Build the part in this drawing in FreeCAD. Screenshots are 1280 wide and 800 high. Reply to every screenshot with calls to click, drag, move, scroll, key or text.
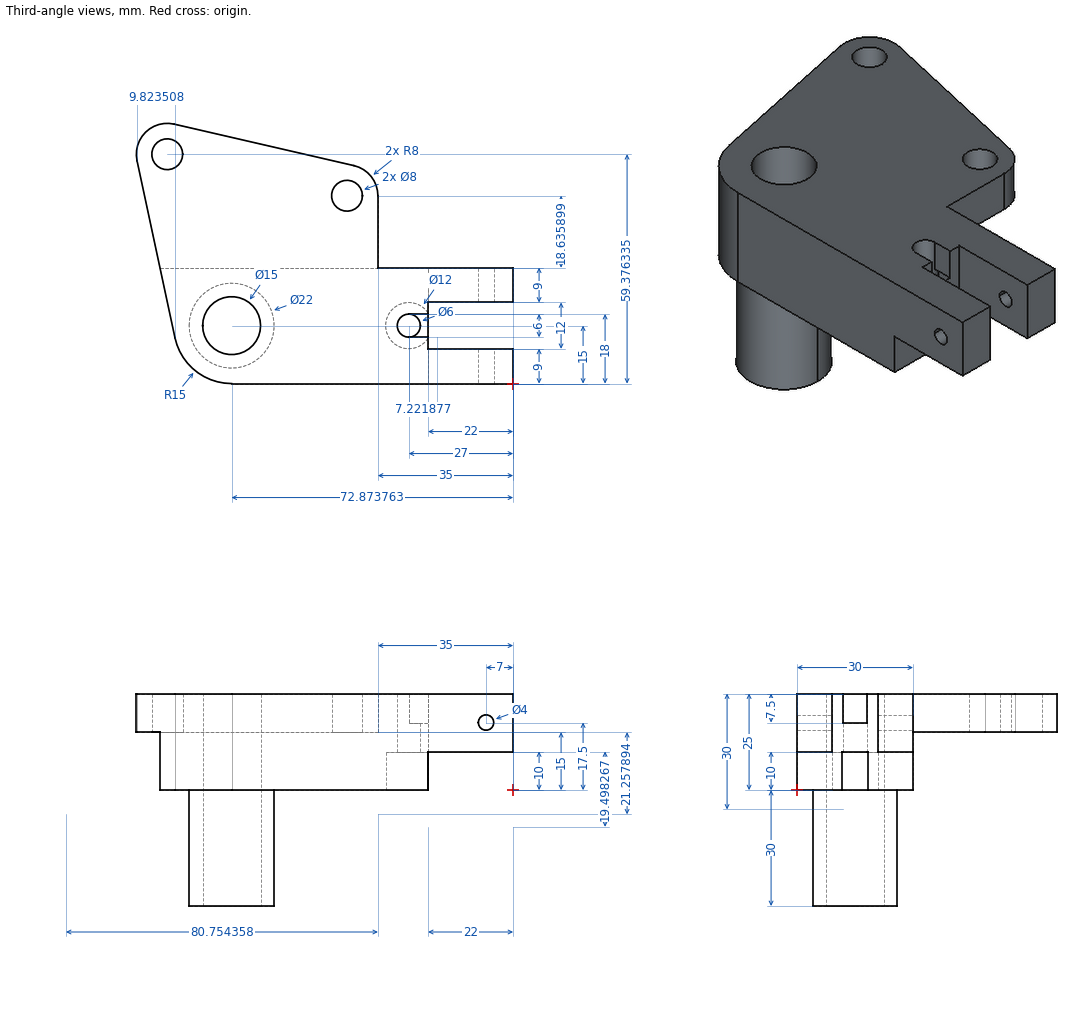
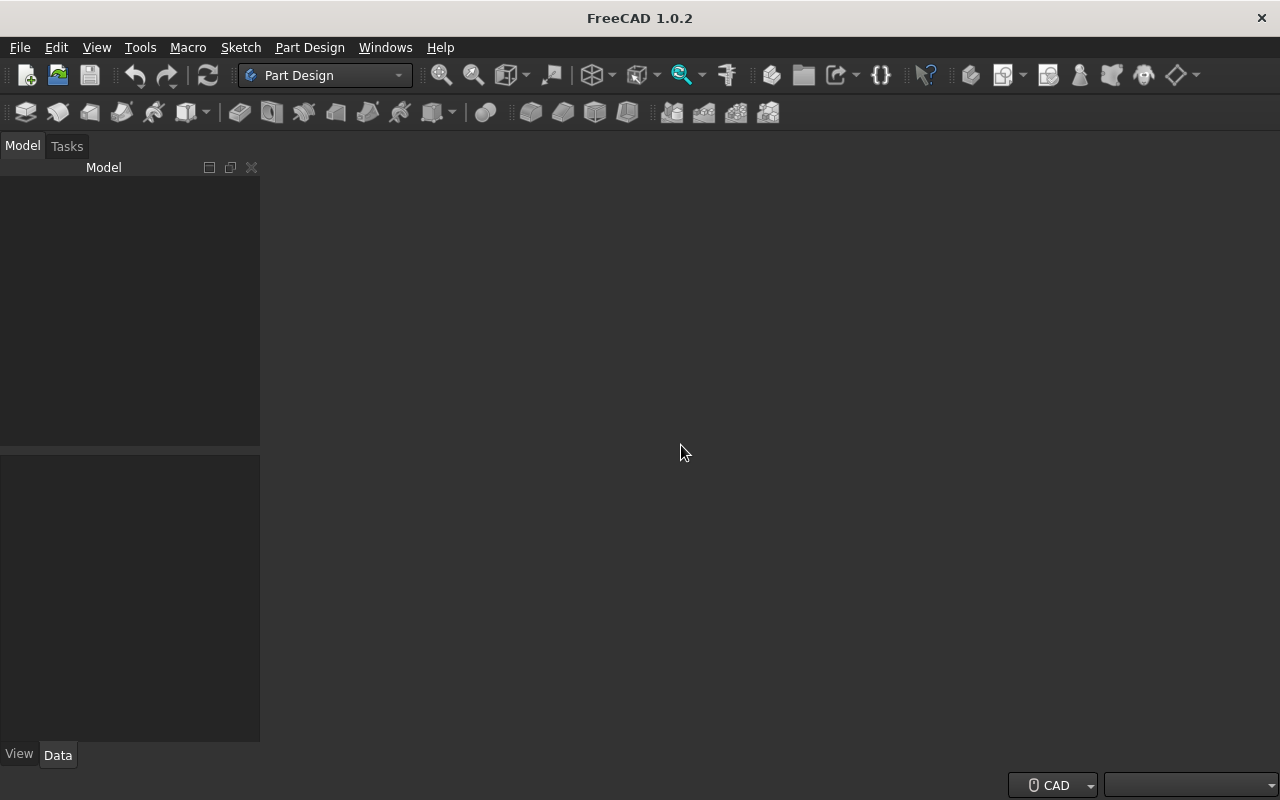
key(ctrl+n)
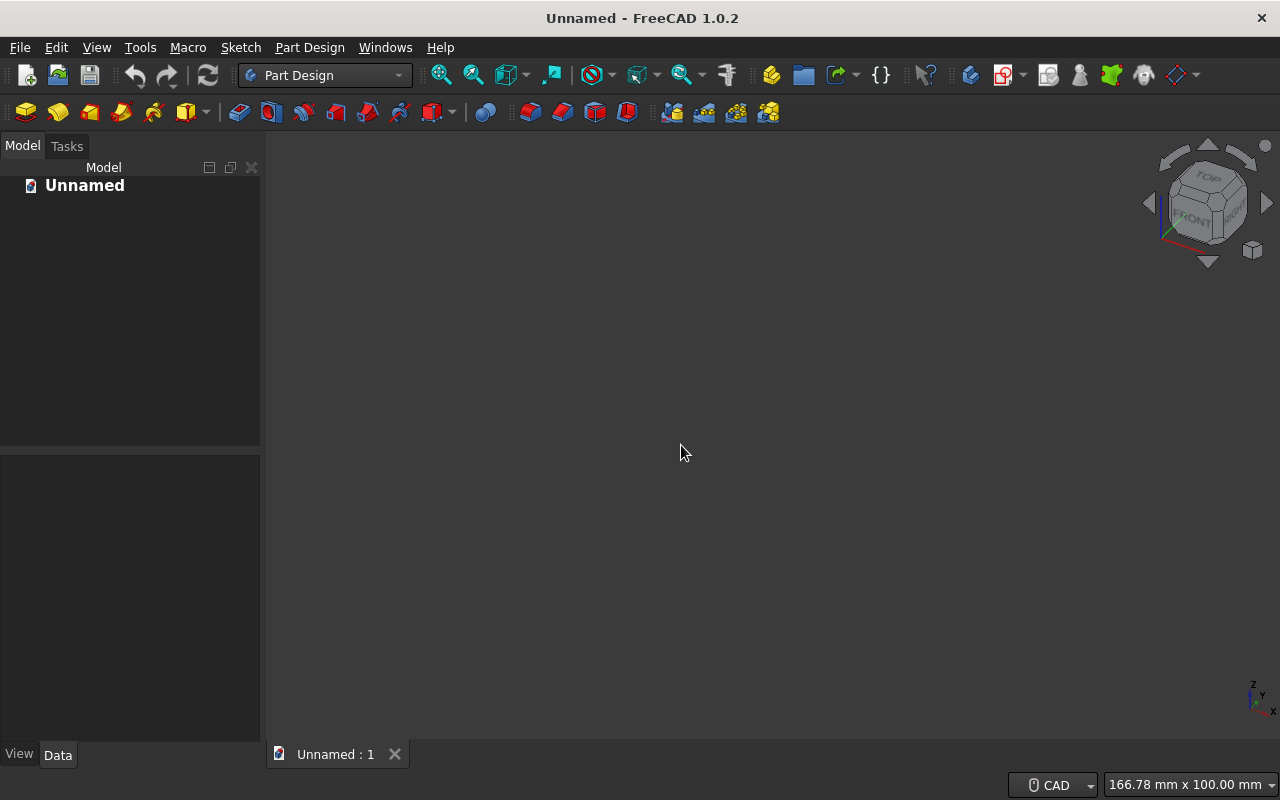
click(1004, 76)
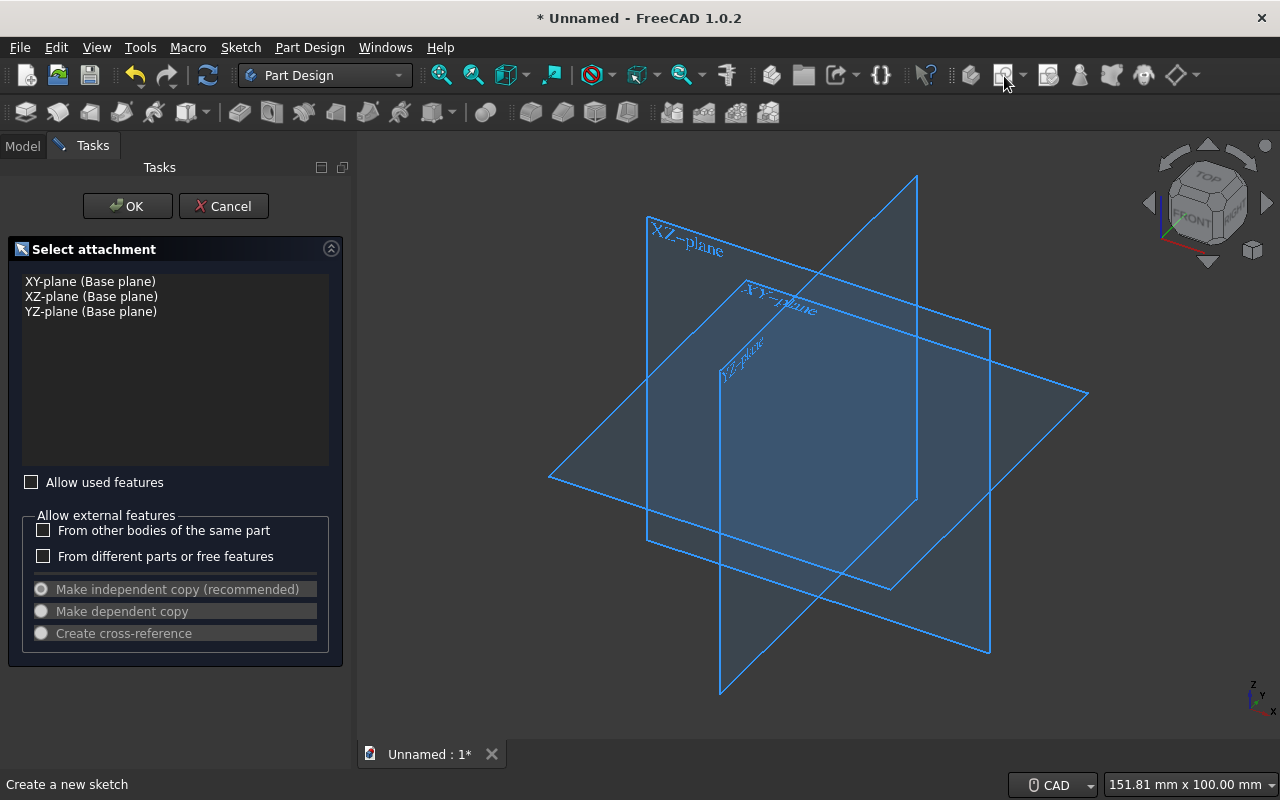
click(82, 282)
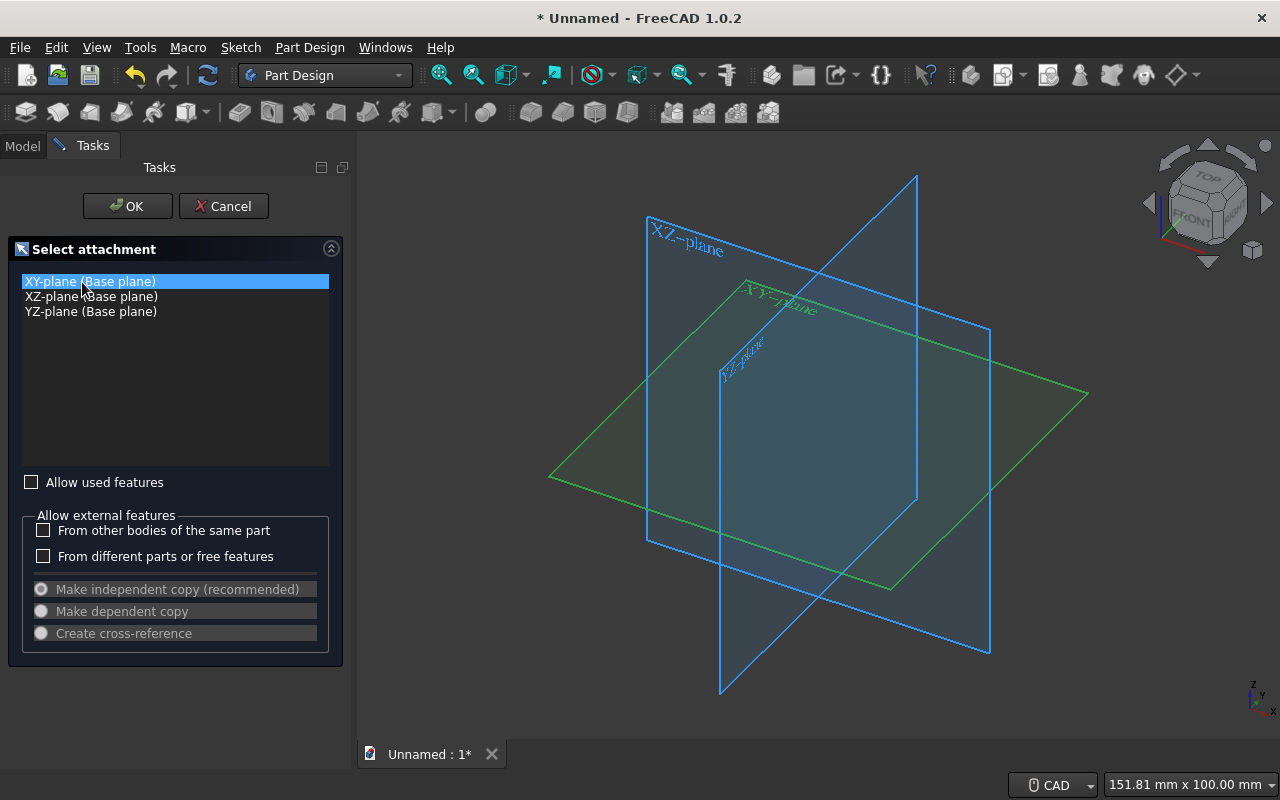
click(128, 206)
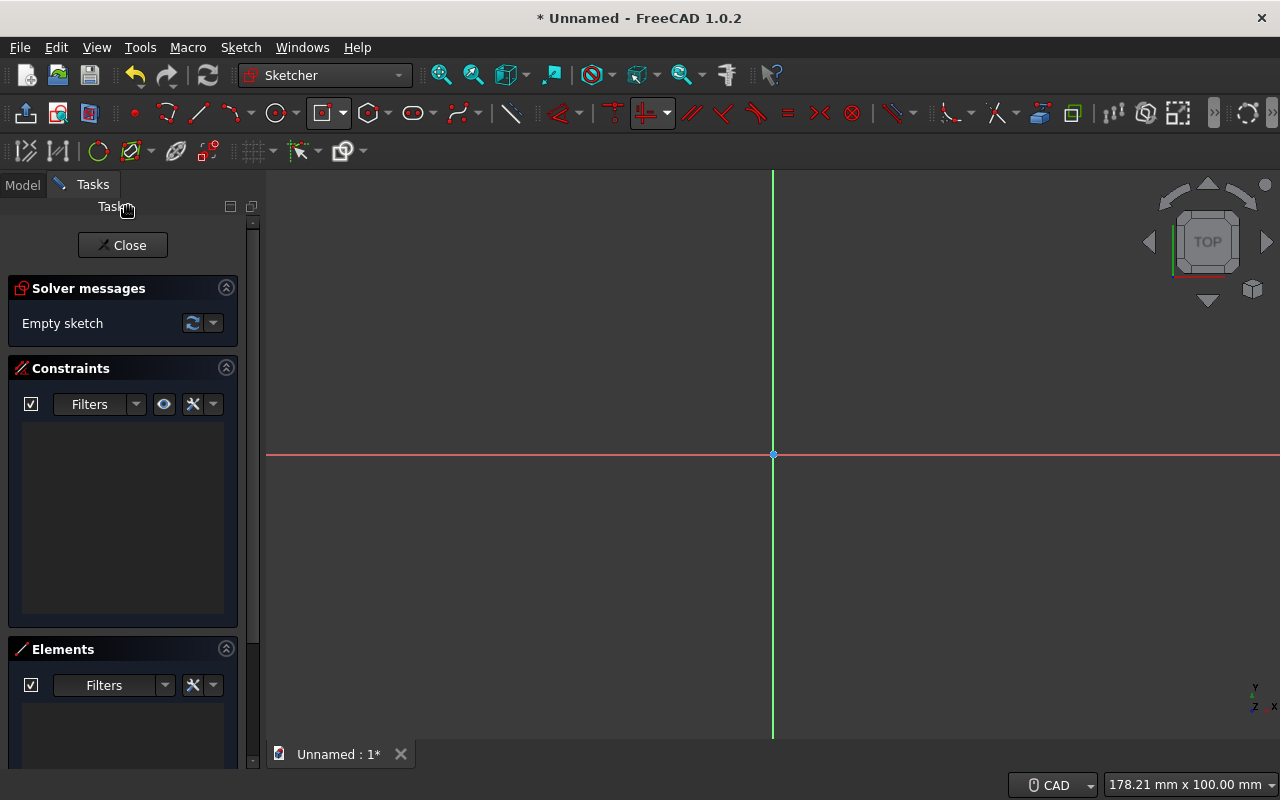
scroll(1115, 711, down, 2)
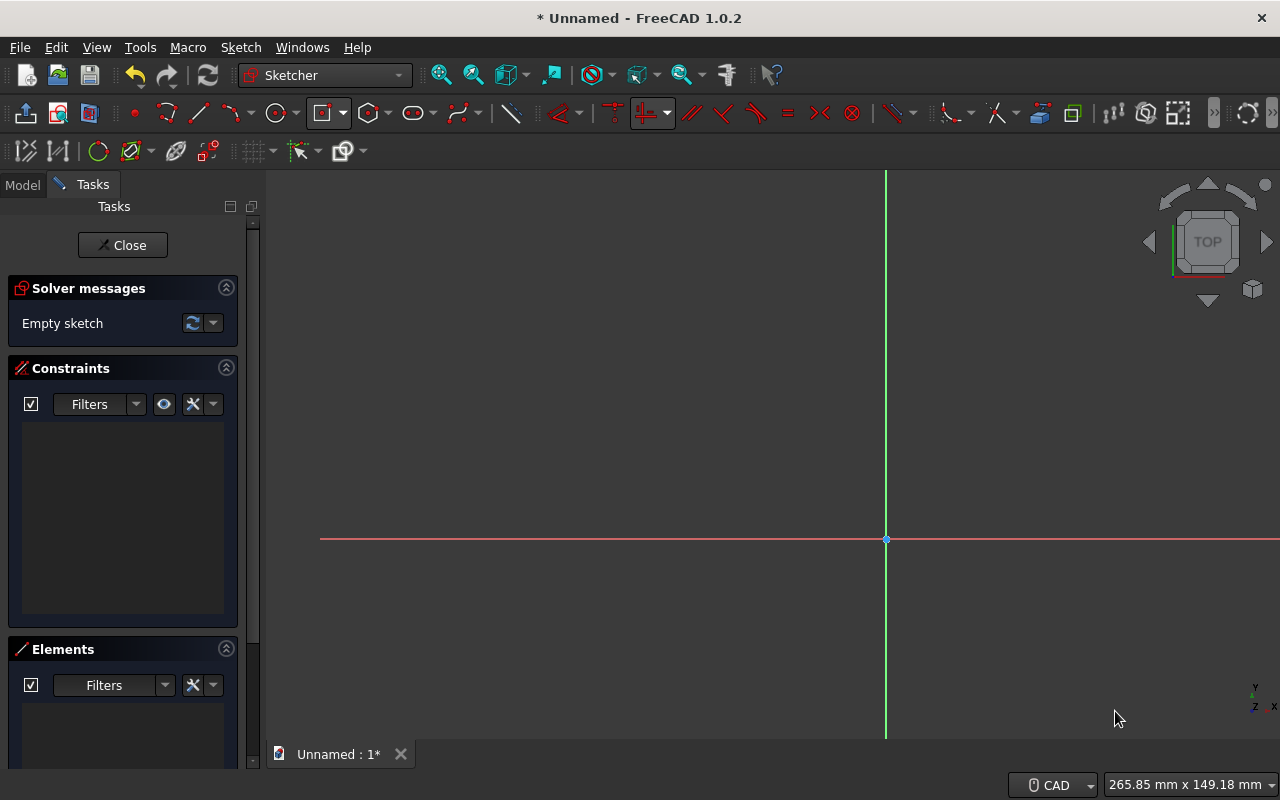
scroll(692, 323, up, 2)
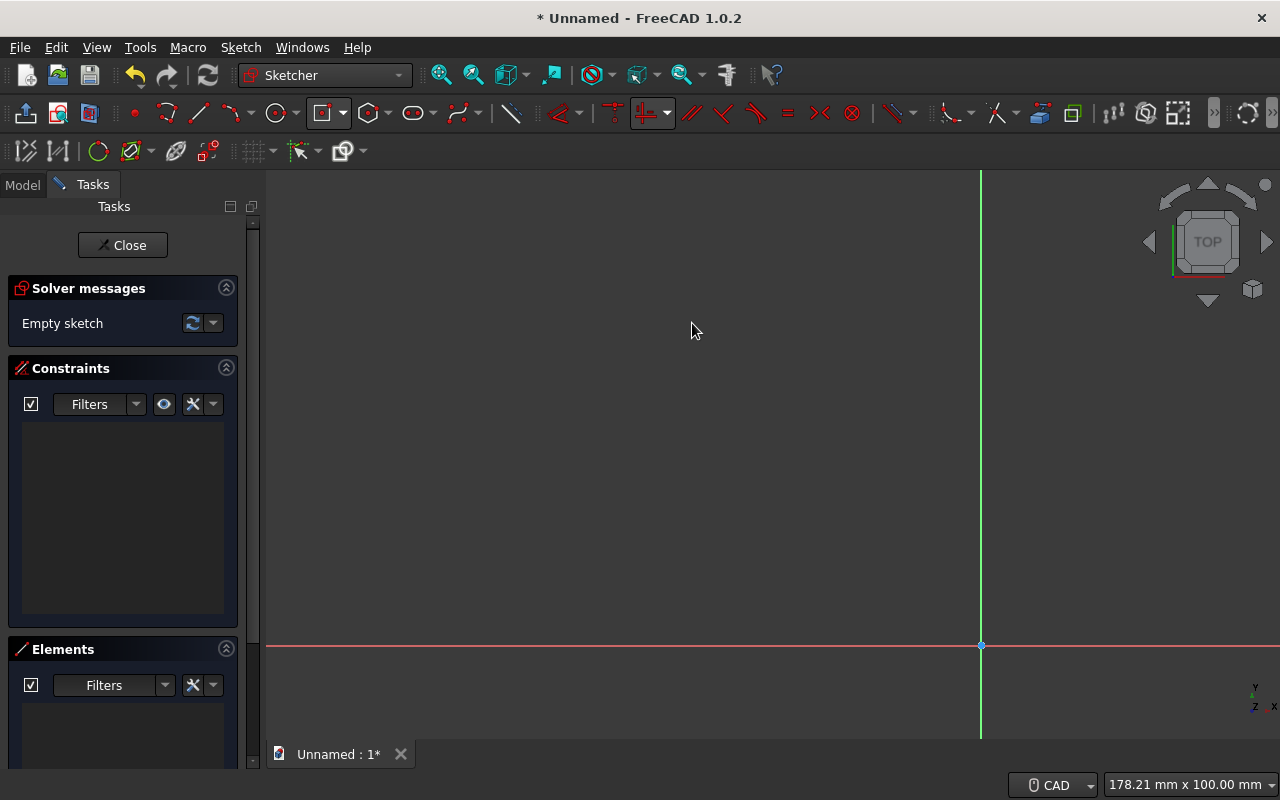
click(168, 114)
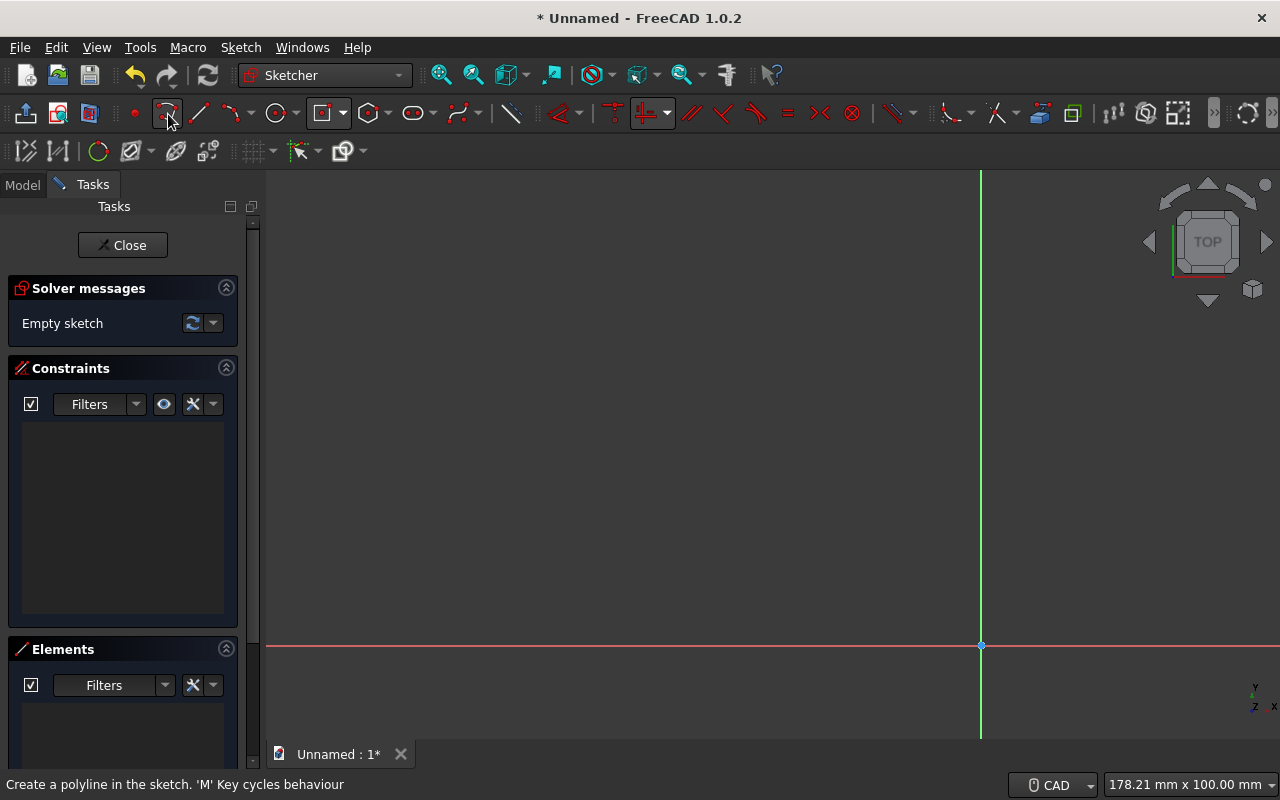
click(567, 646)
click(981, 646)
click(972, 594)
click(856, 594)
click(856, 526)
click(981, 526)
click(972, 475)
click(782, 475)
click(782, 369)
right_click(782, 369)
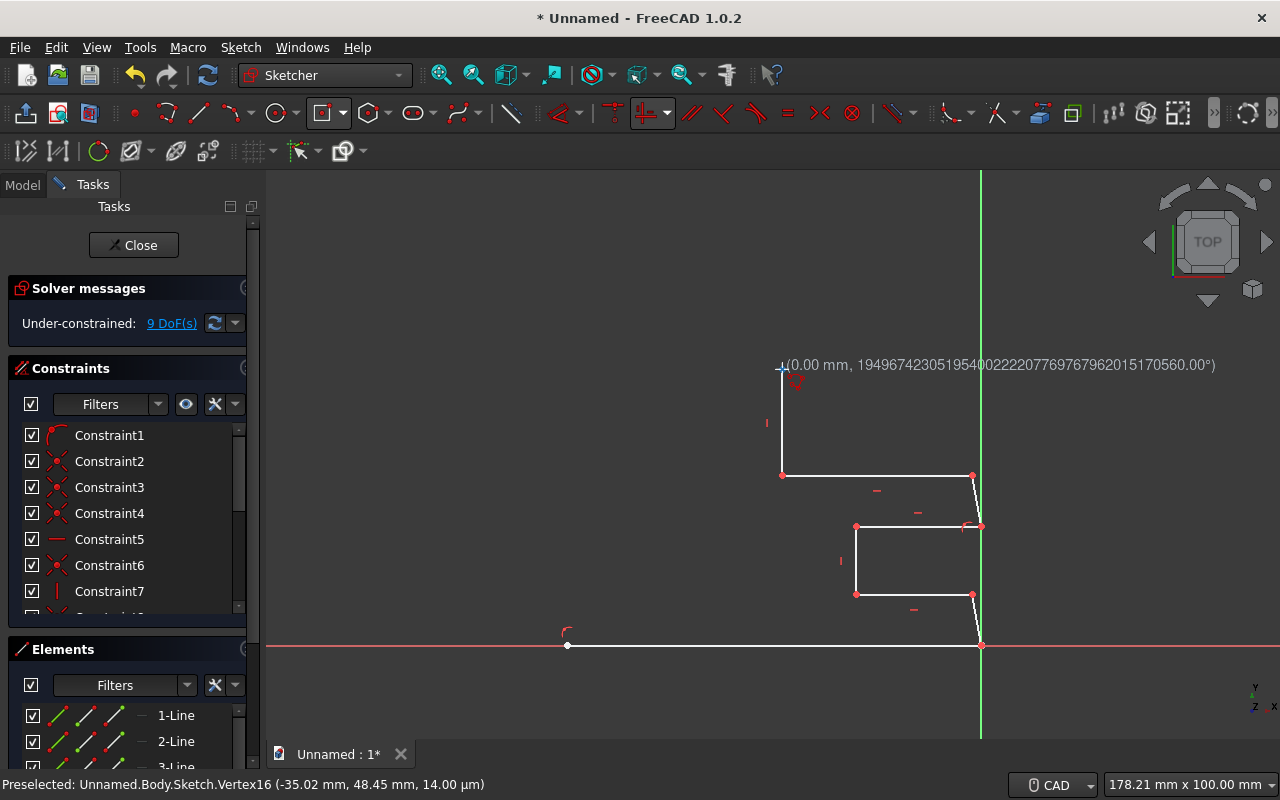
click(200, 114)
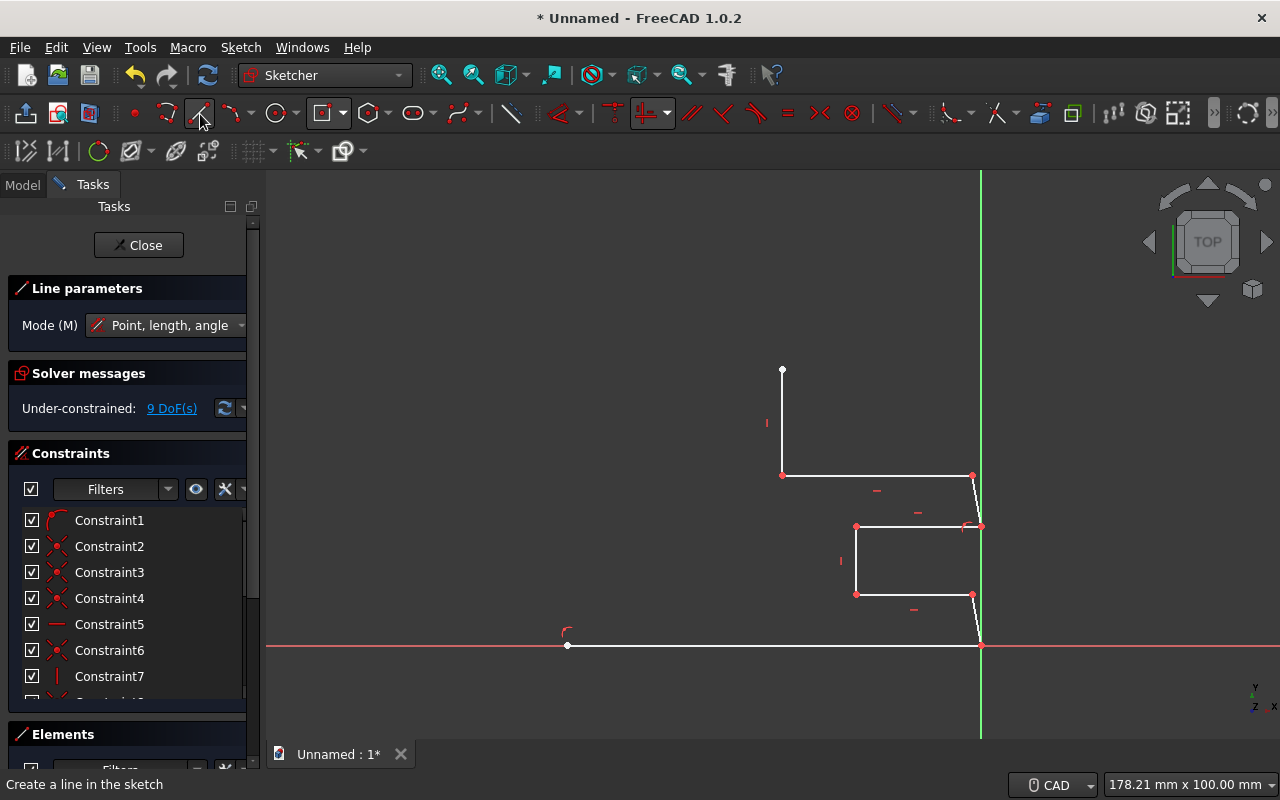
click(747, 325)
click(482, 263)